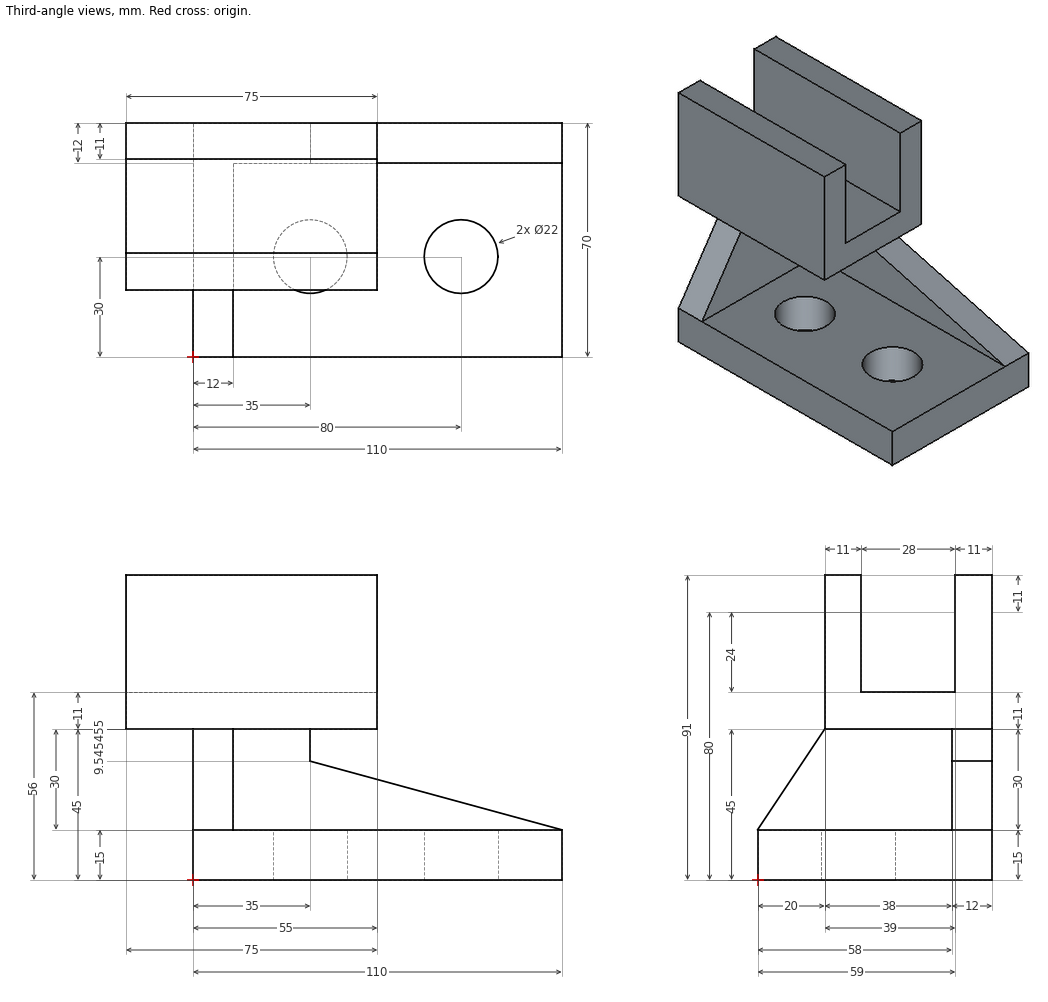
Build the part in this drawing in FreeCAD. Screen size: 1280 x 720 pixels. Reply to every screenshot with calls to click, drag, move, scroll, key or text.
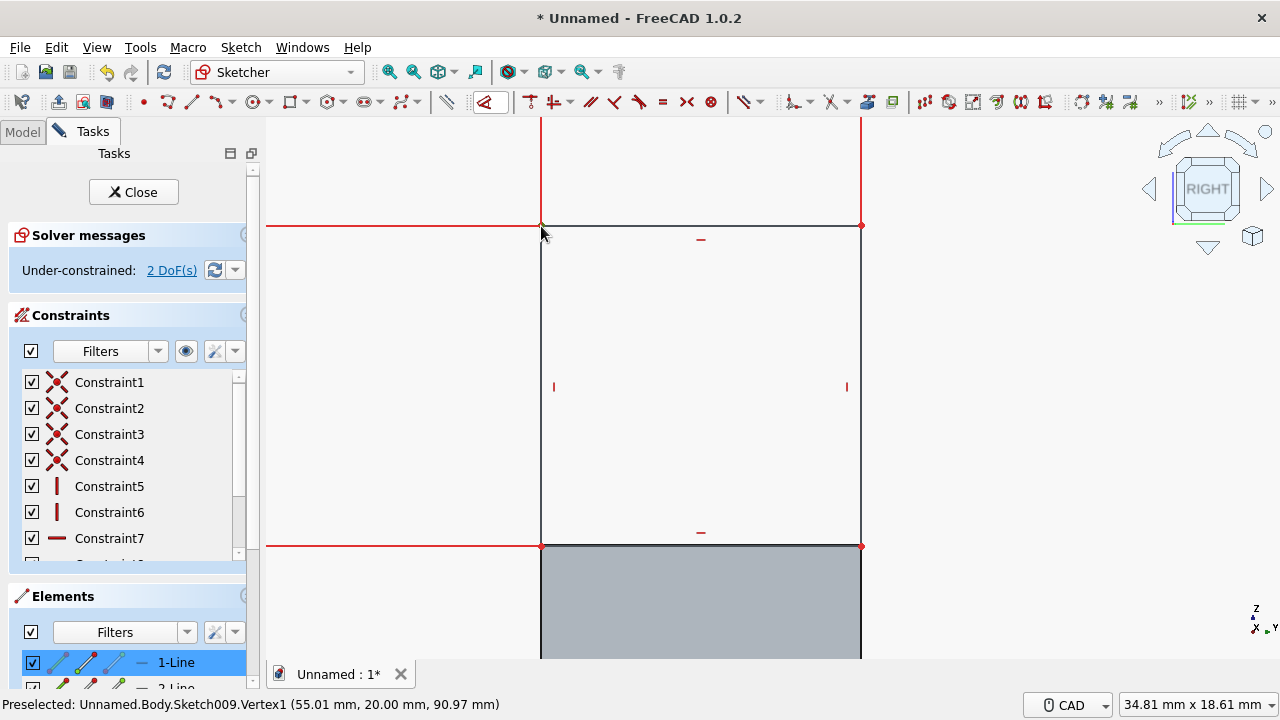
key(l)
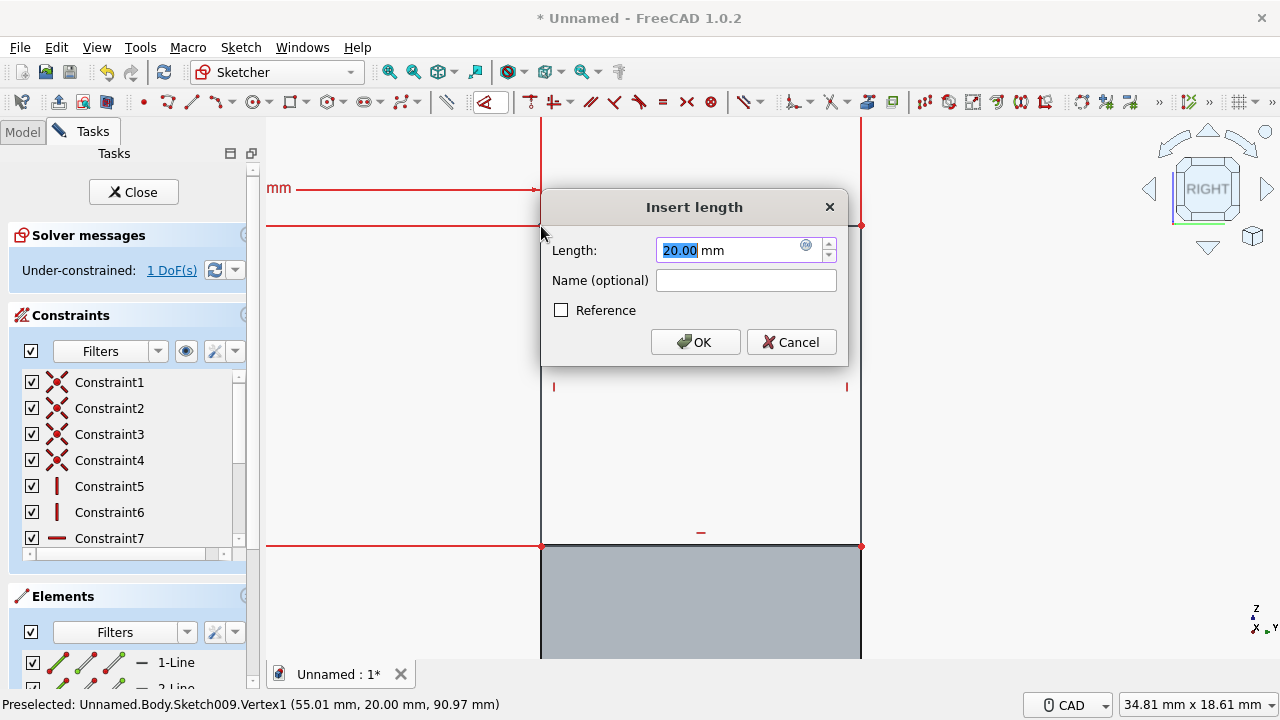
text(20)
key(Return)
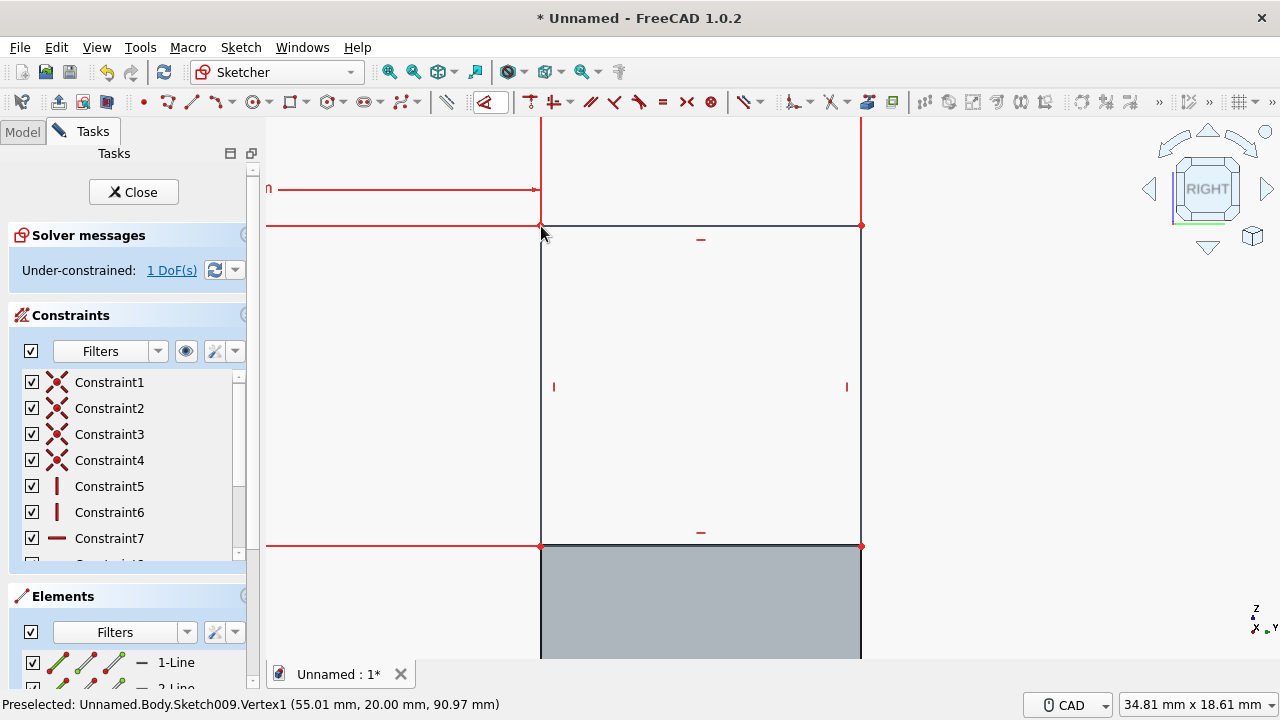
click(541, 226)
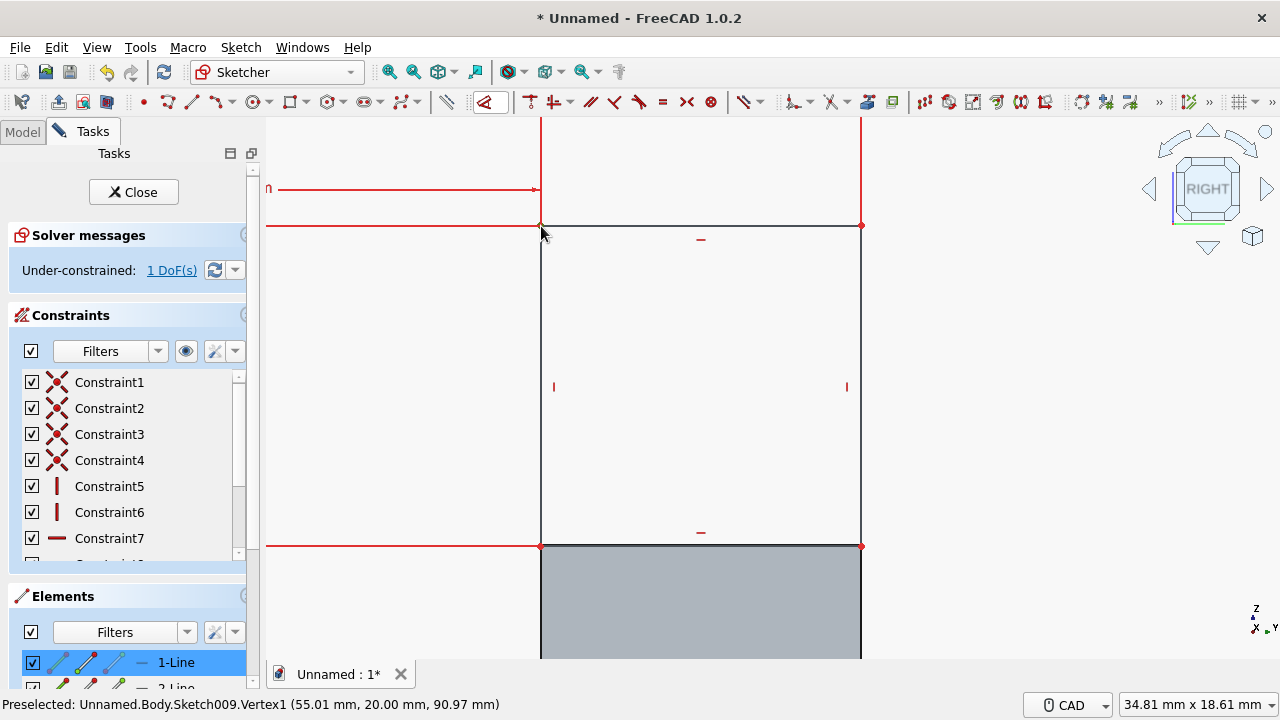
key(i)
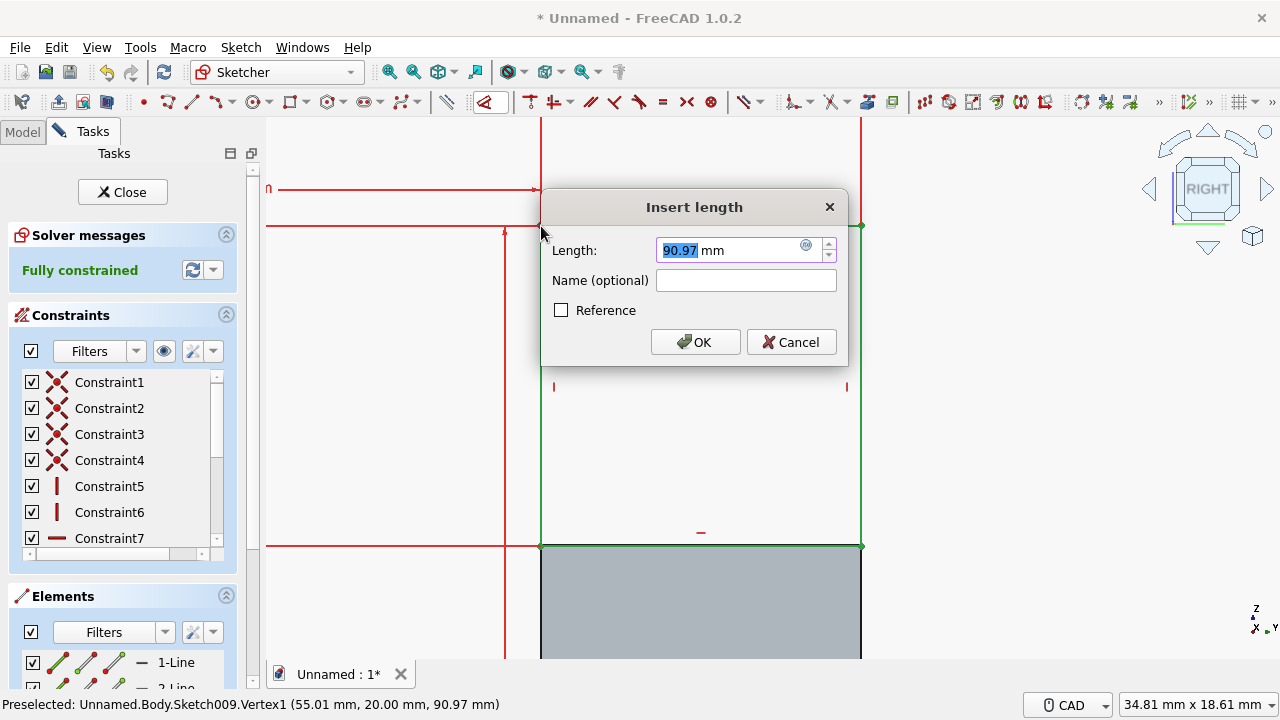
text(91)
key(Return)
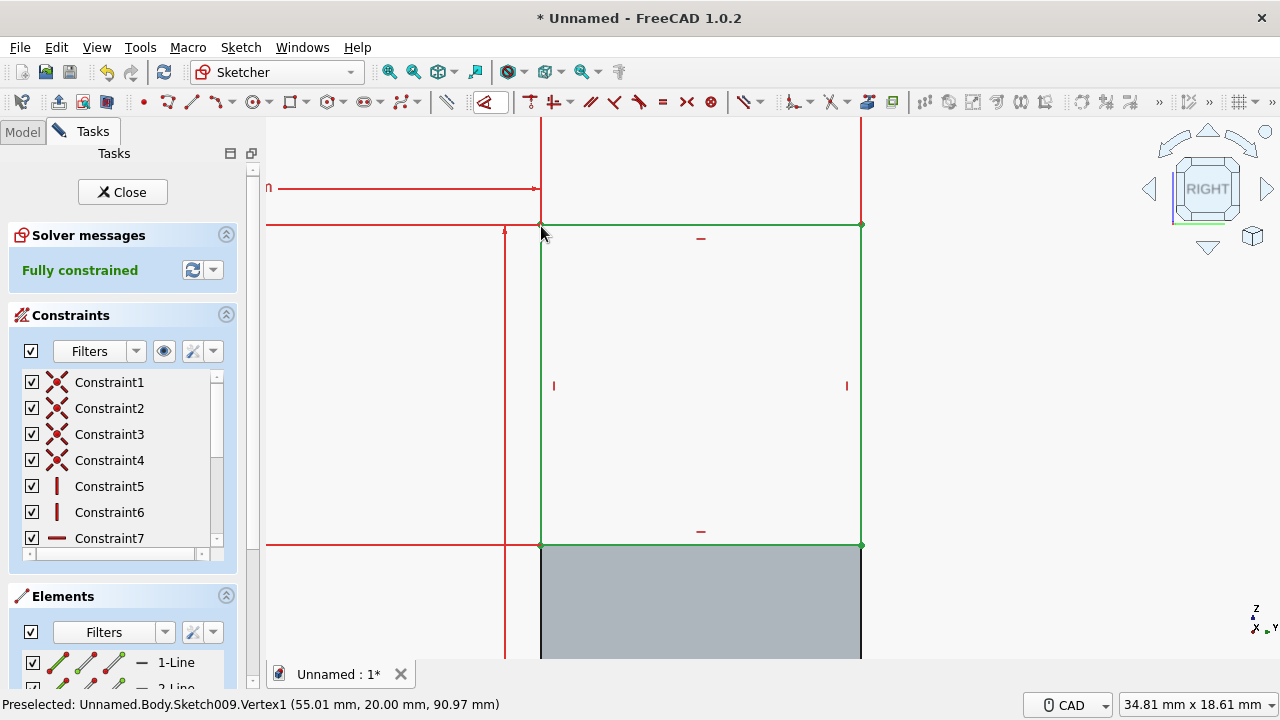
click(123, 192)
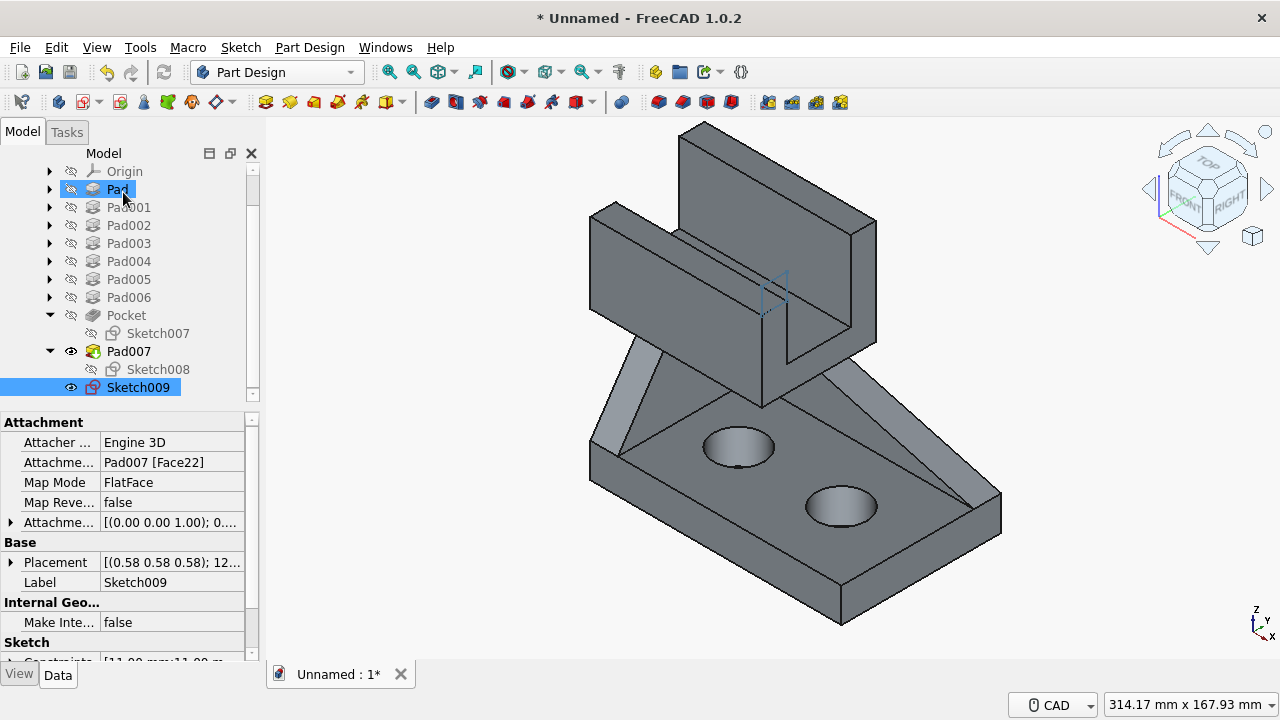
click(266, 102)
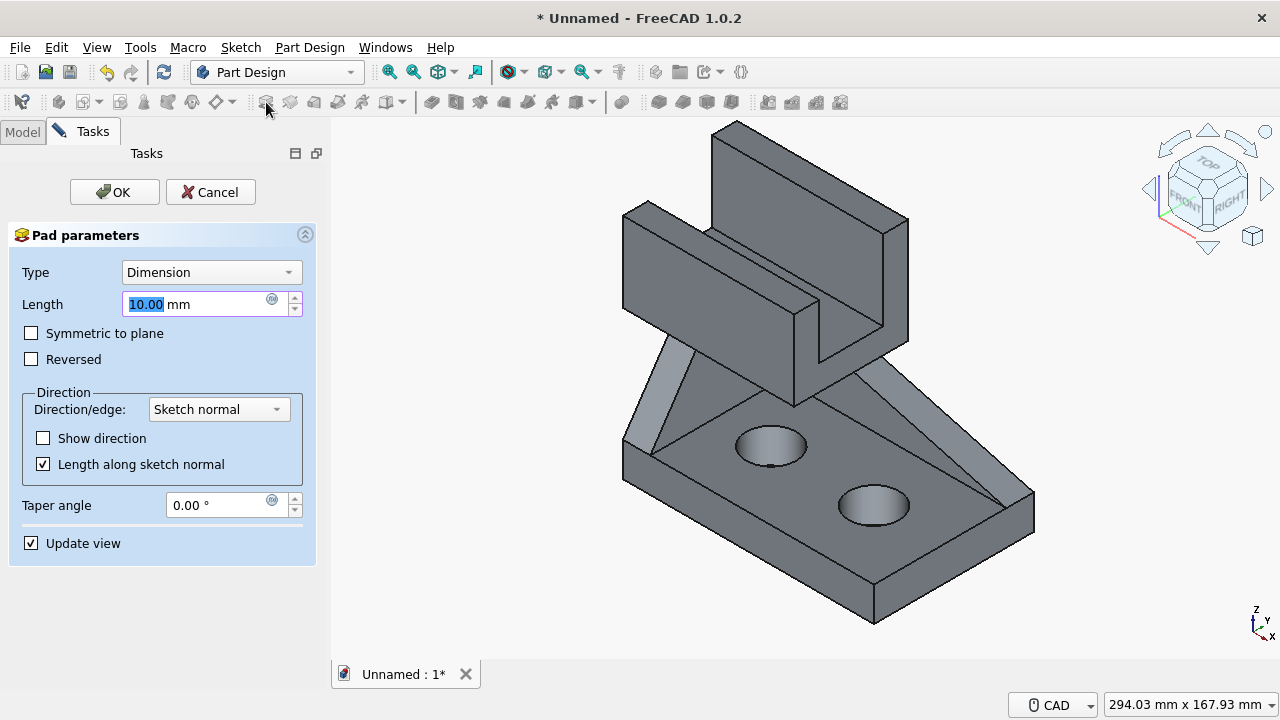
text(75)
key(Tab)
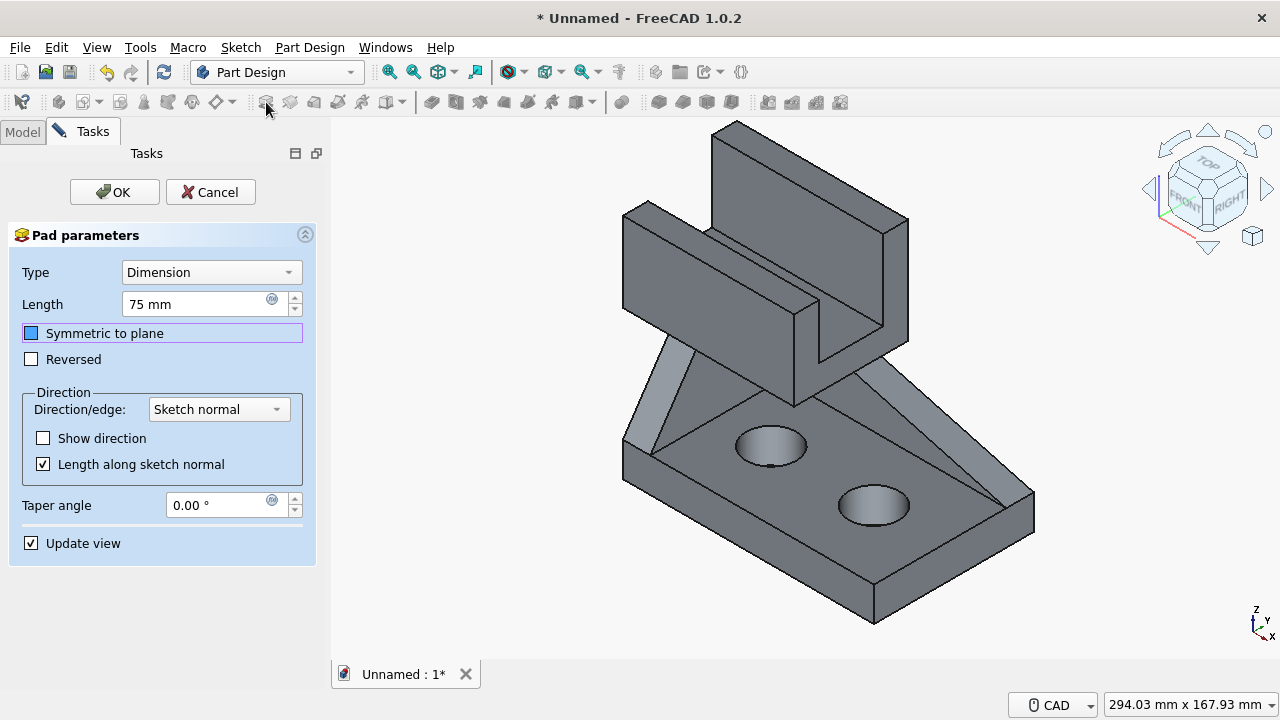
click(30, 359)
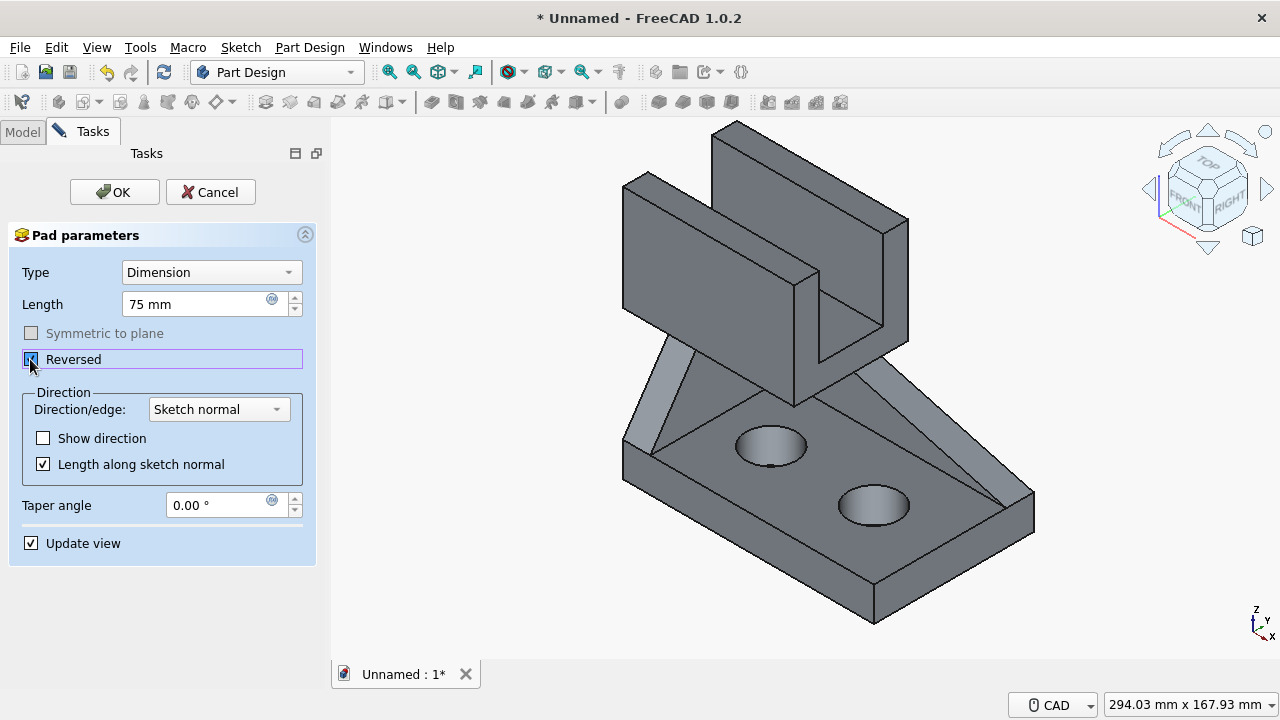
click(115, 192)